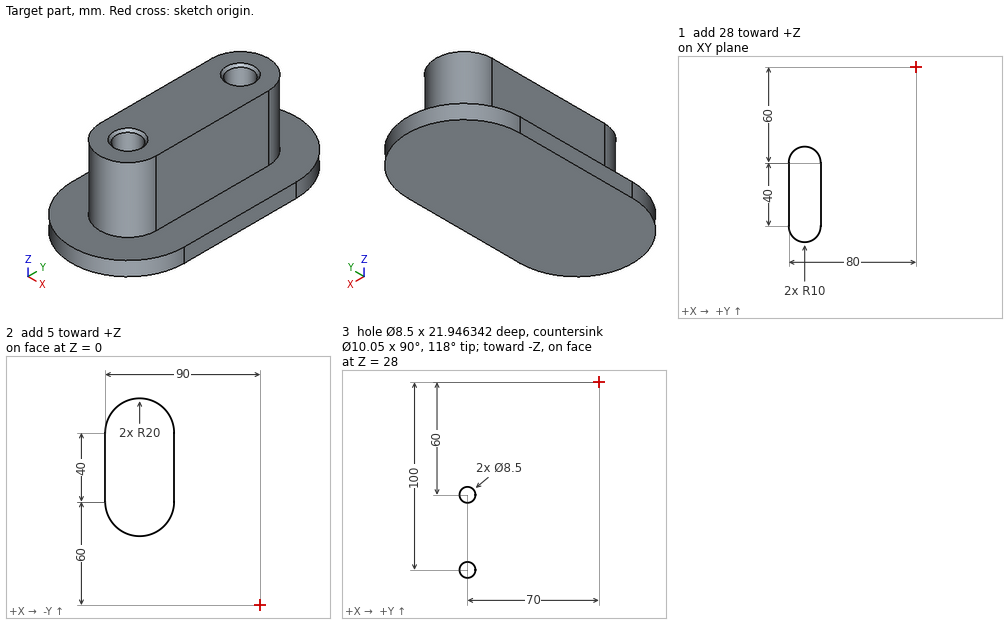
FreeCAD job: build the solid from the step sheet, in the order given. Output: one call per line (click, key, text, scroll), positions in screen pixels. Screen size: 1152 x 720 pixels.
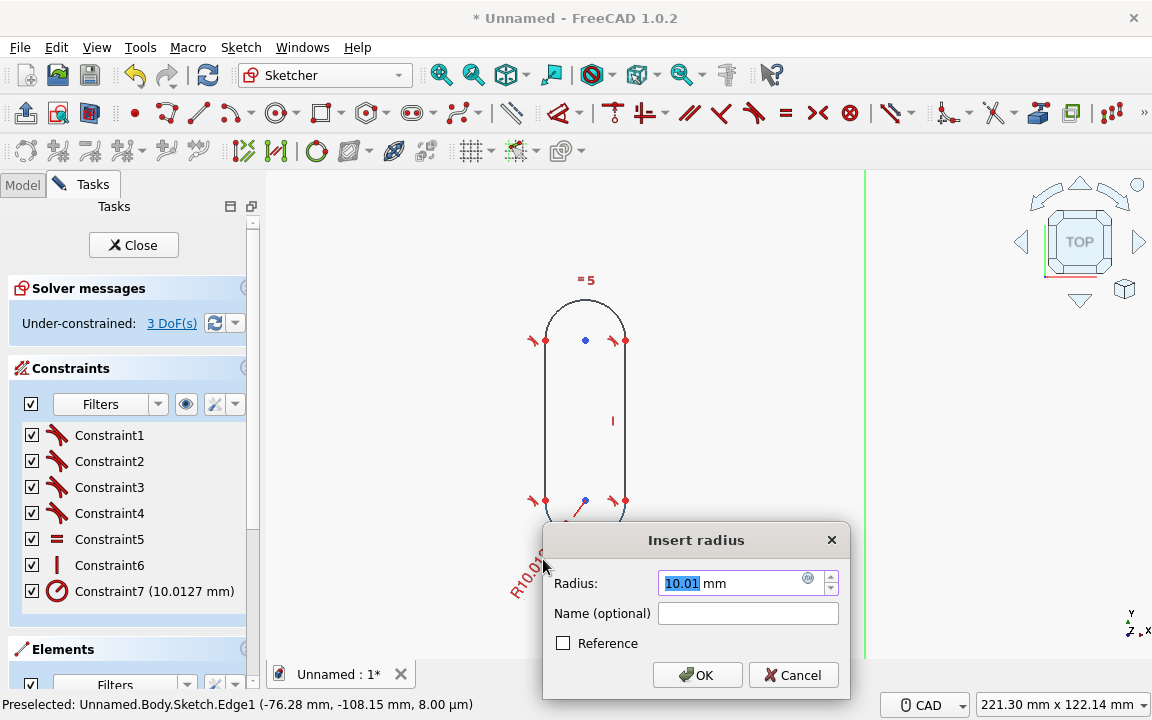
text(10)
key(Return)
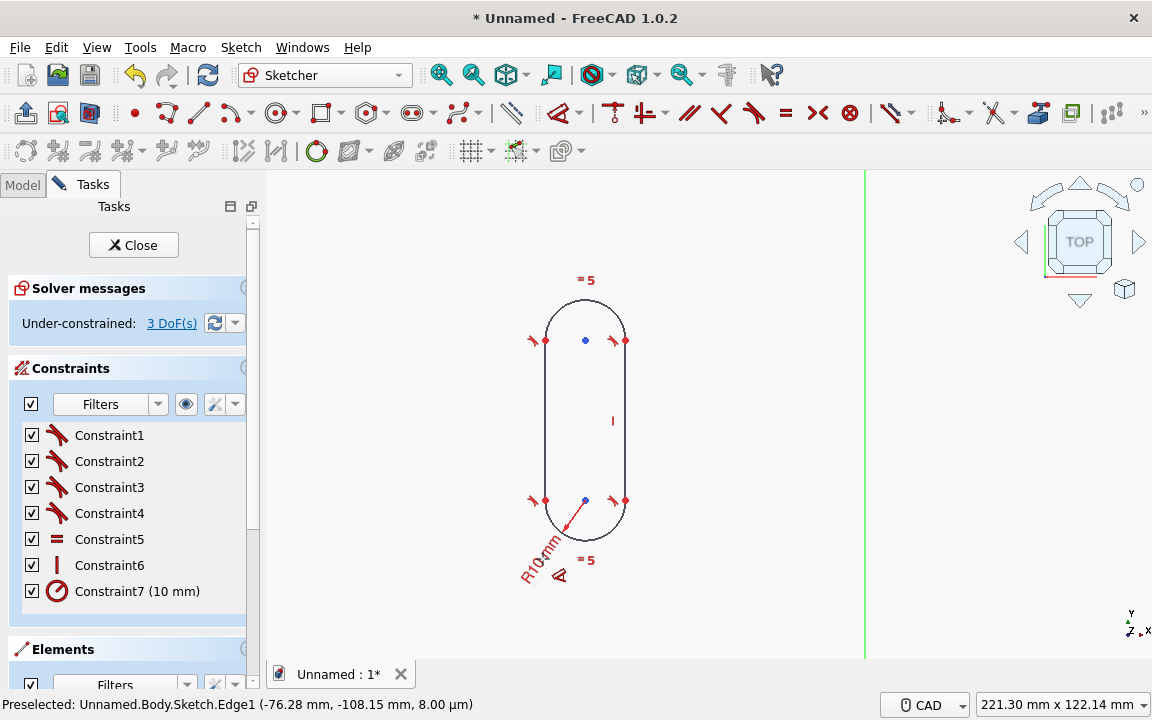
click(545, 452)
click(511, 420)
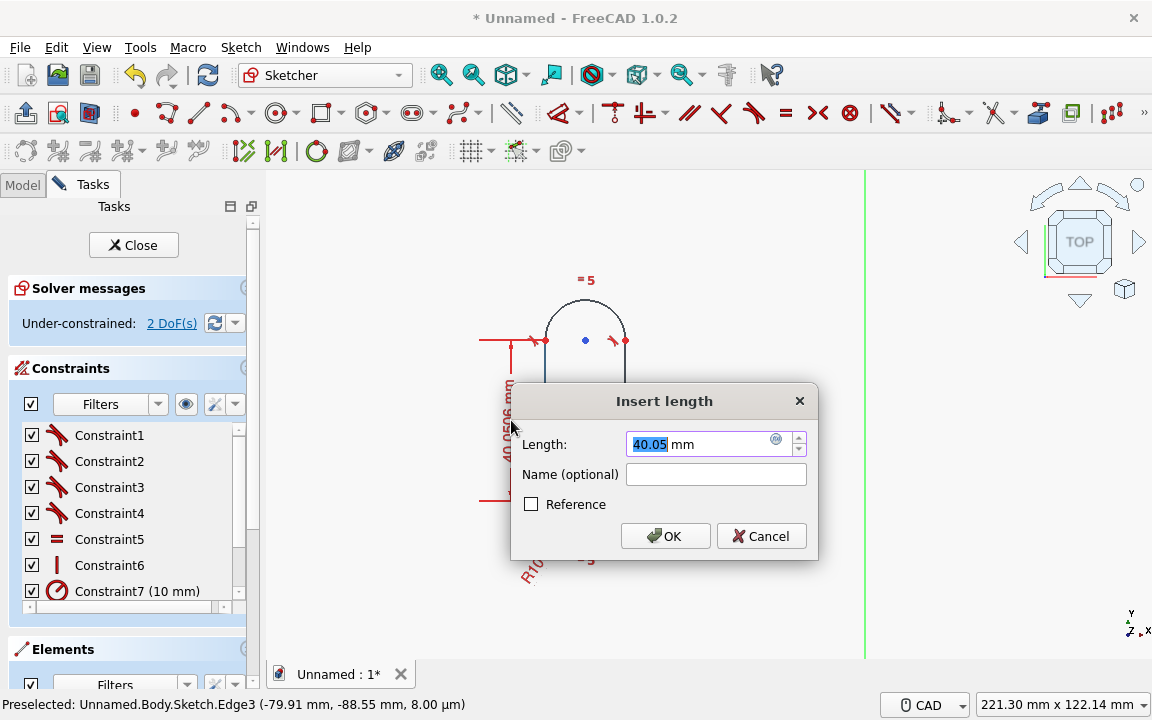
text(40)
key(Return)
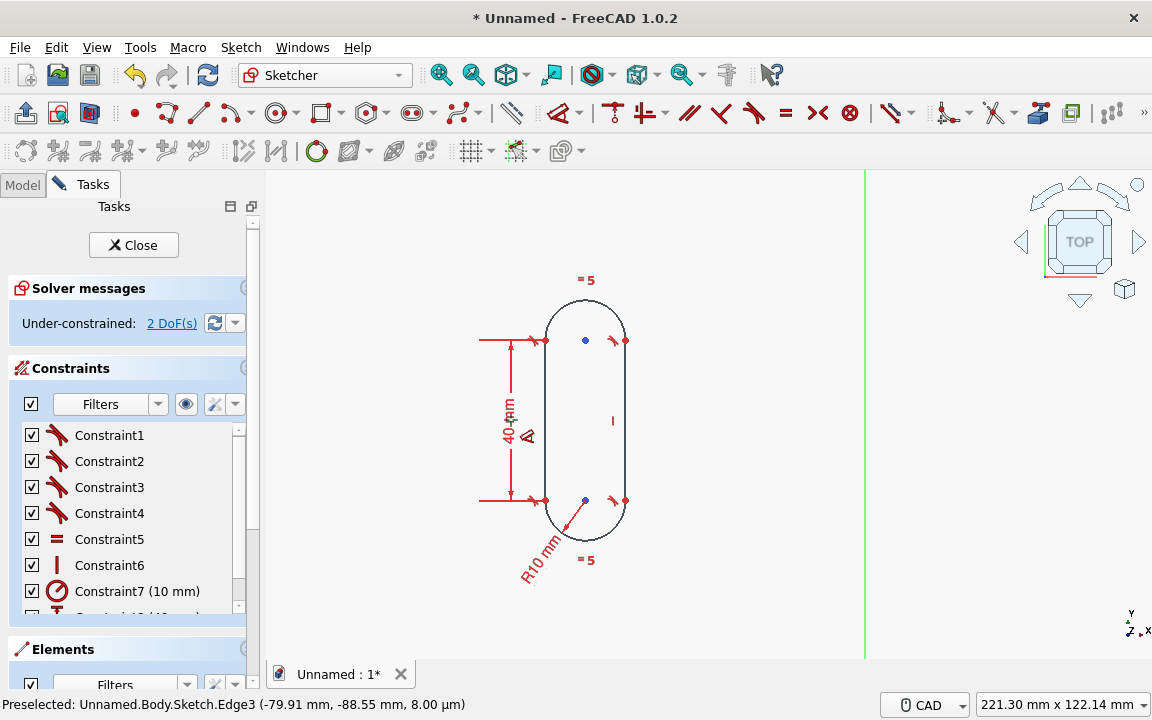
click(545, 501)
click(705, 535)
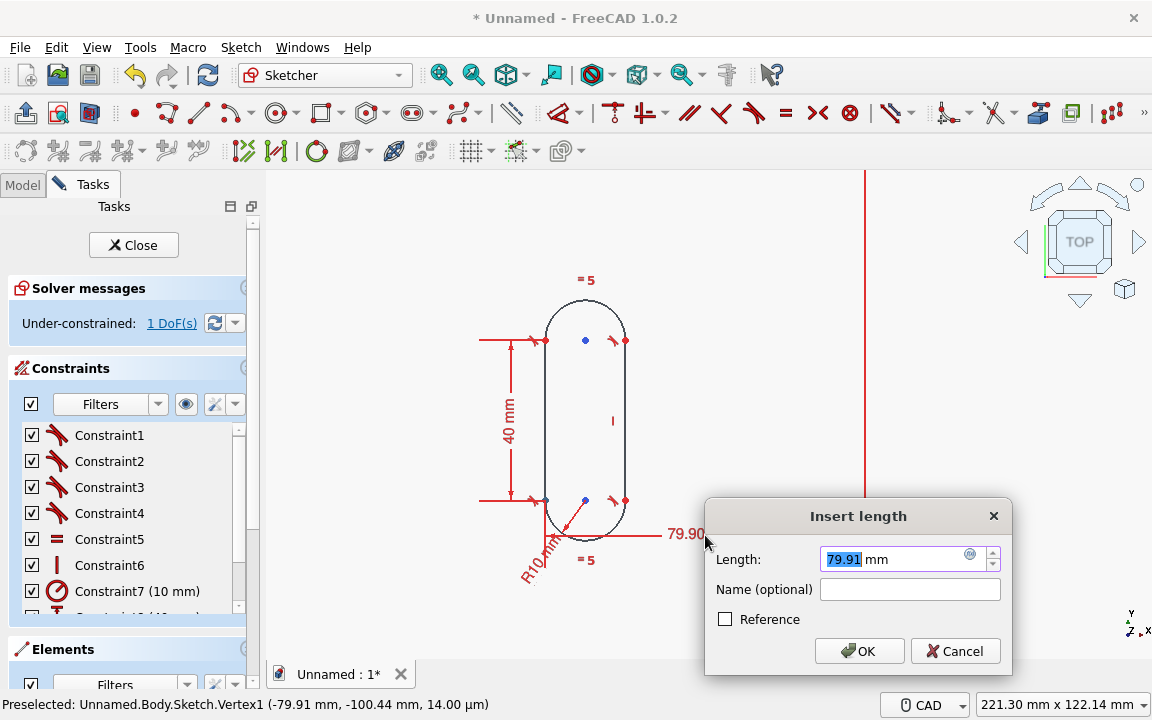
text(80)
key(Return)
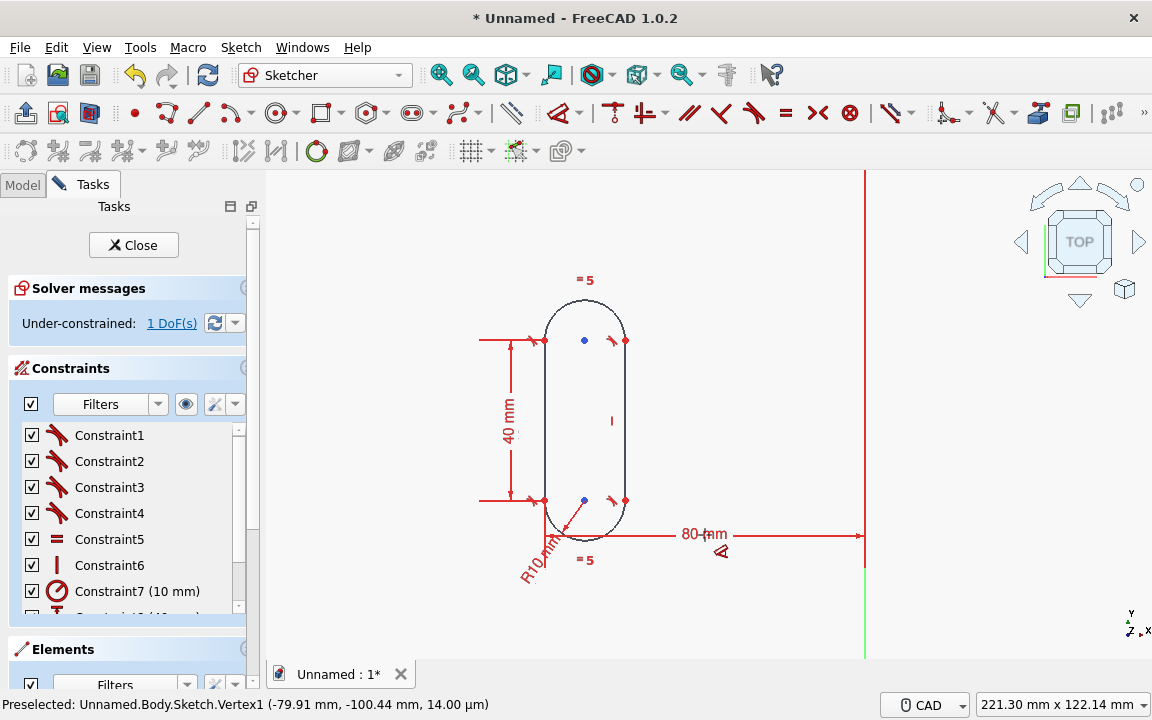
click(625, 340)
click(899, 269)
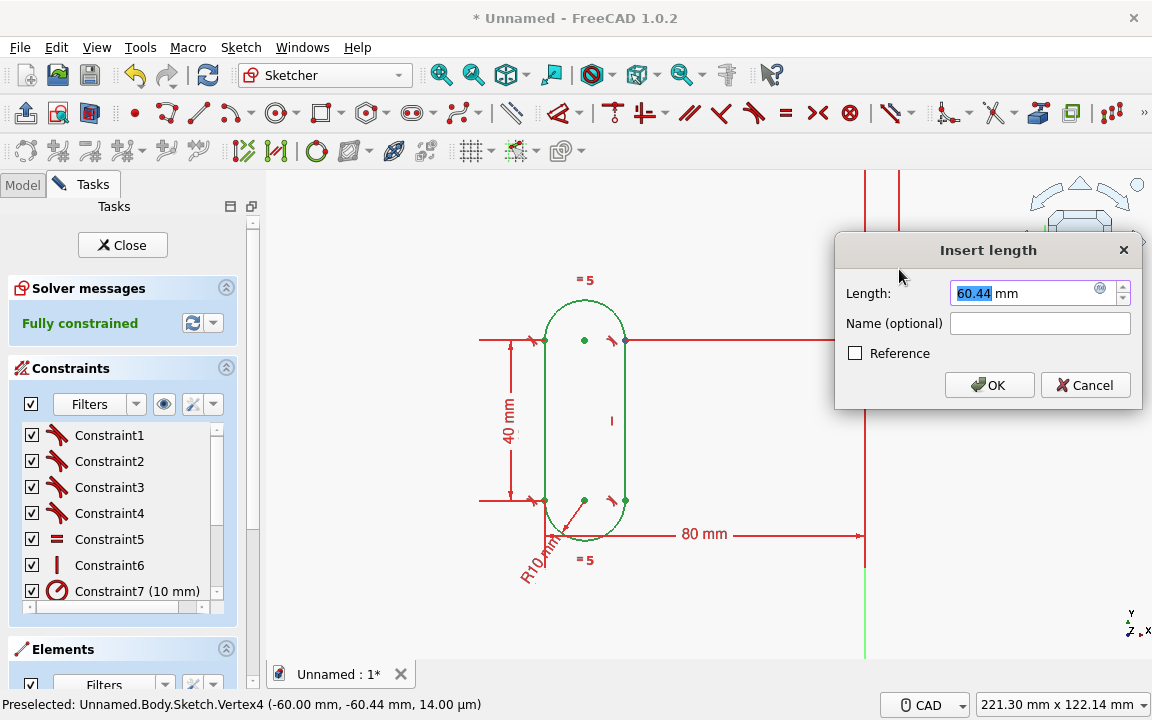
text(60)
key(Return)
key(Escape)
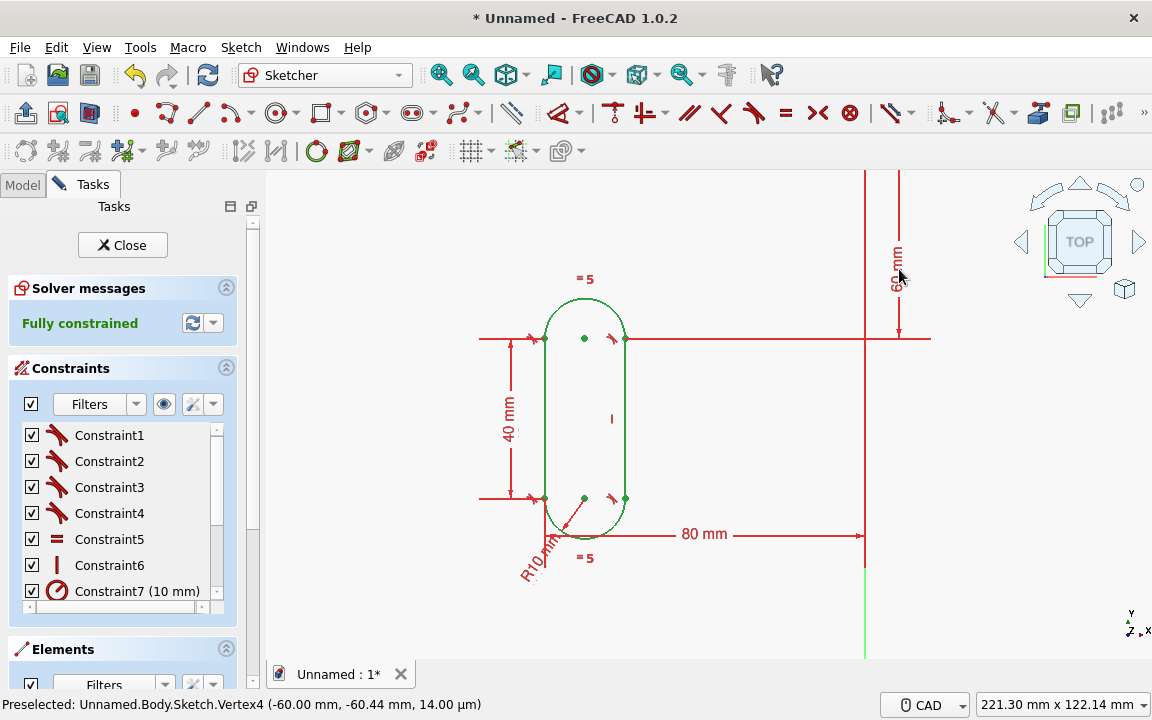
click(123, 245)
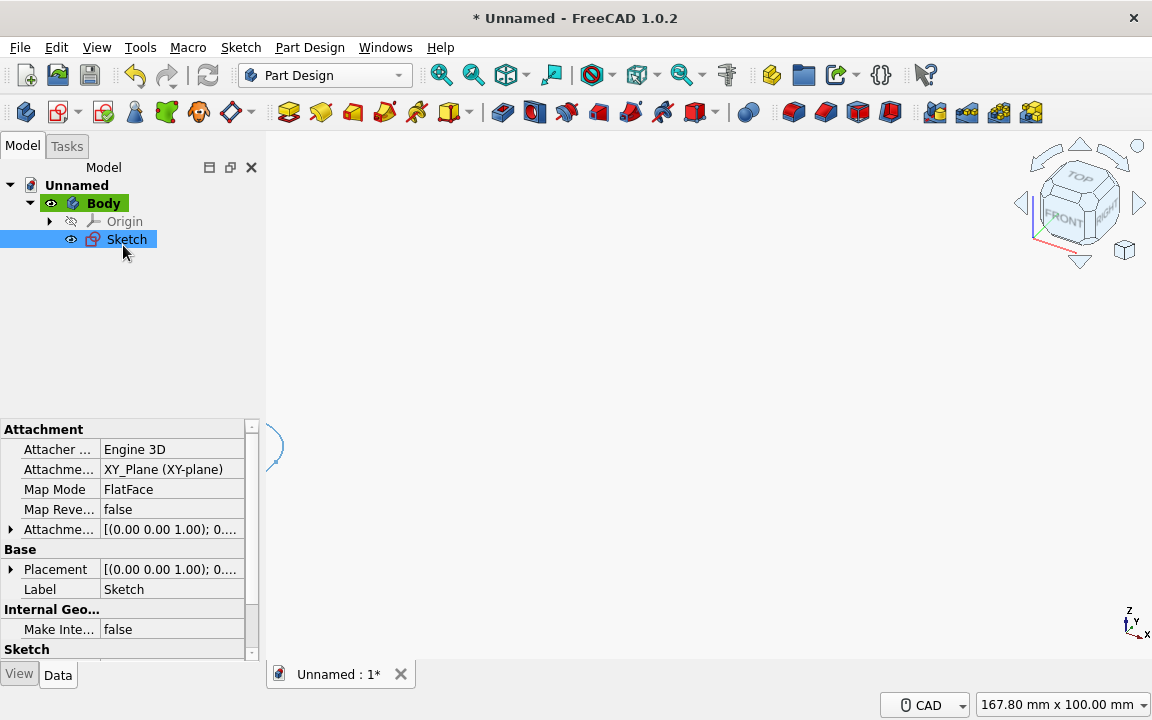
click(290, 112)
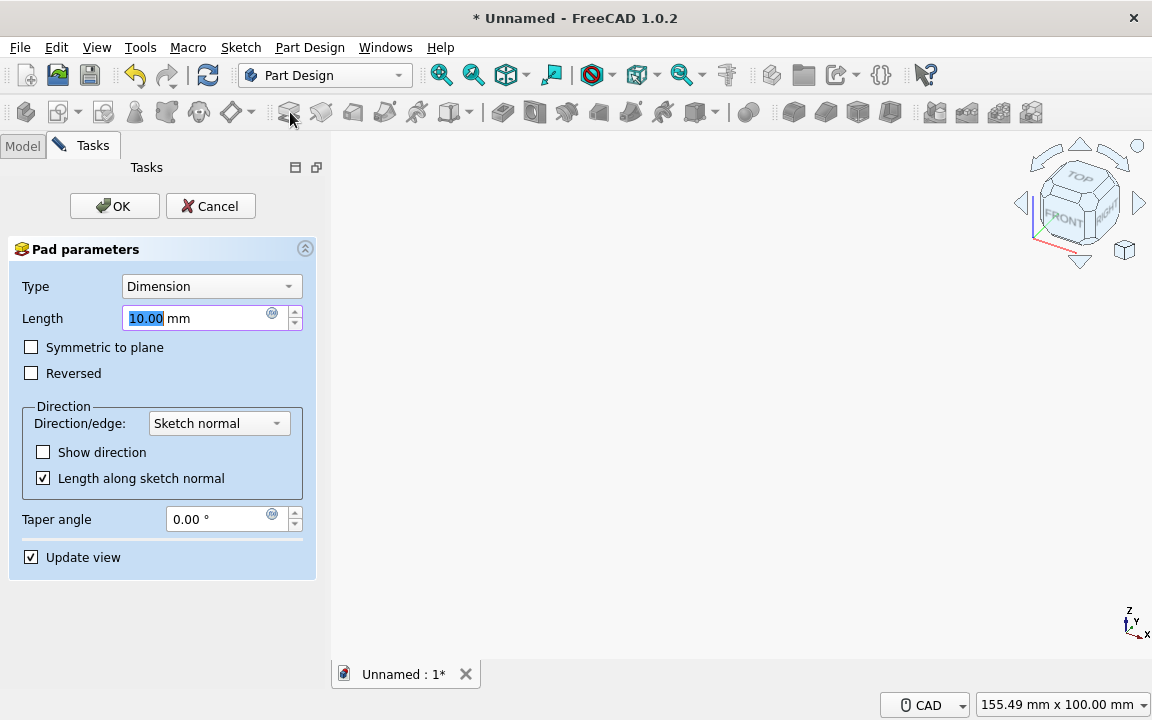
text(28)
key(Tab)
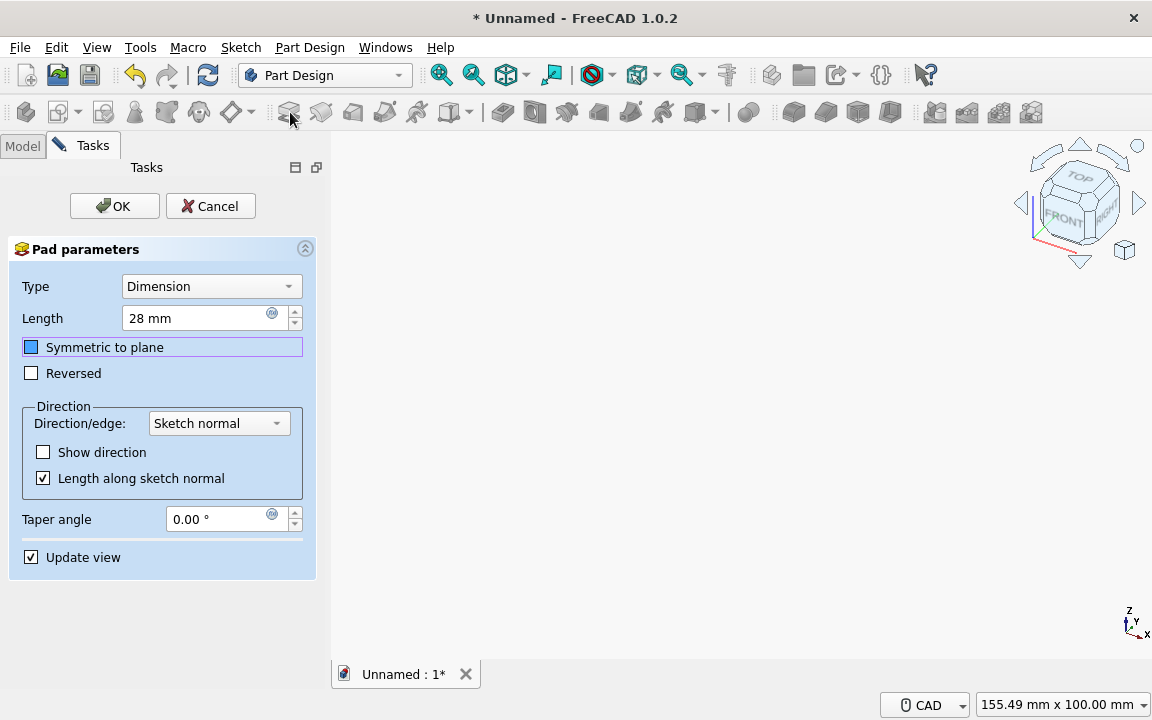
click(115, 206)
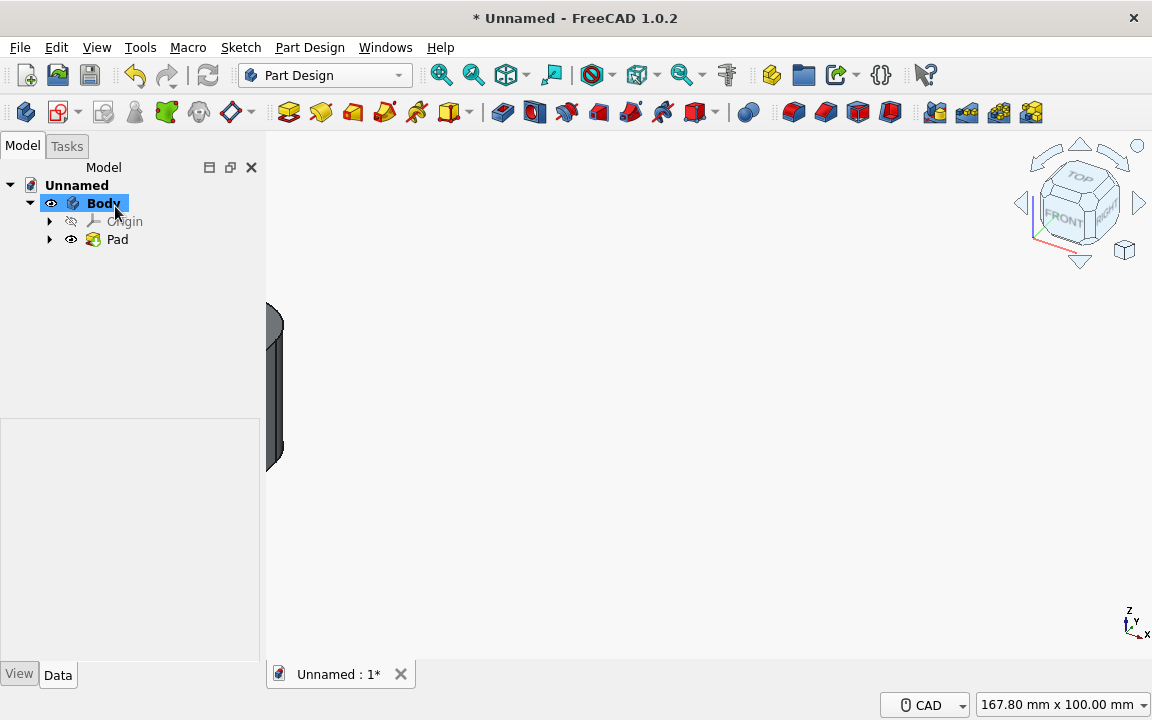
click(442, 76)